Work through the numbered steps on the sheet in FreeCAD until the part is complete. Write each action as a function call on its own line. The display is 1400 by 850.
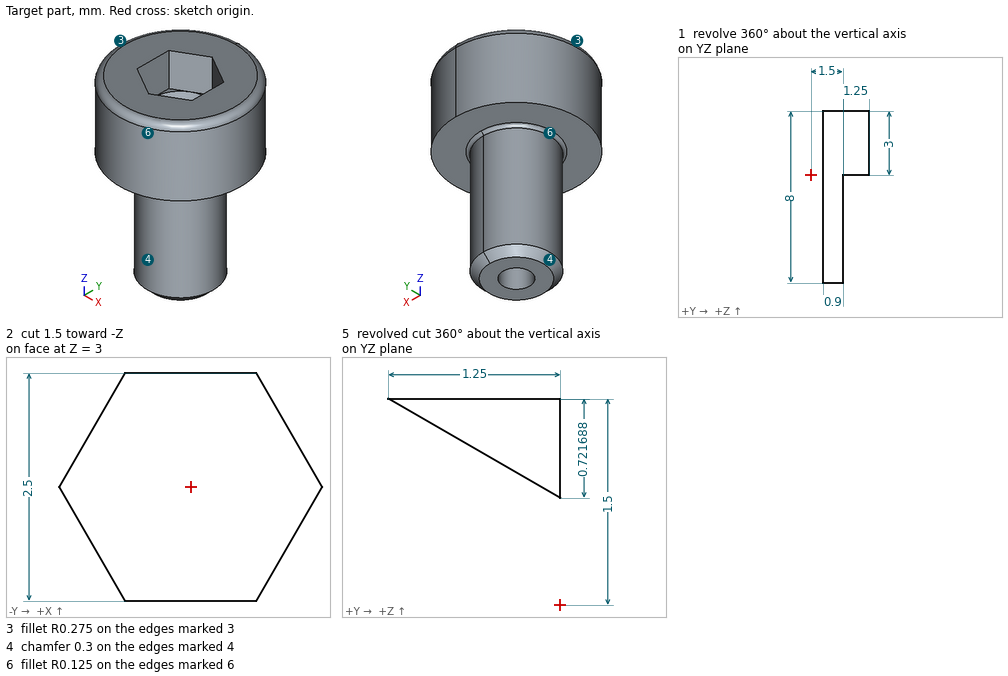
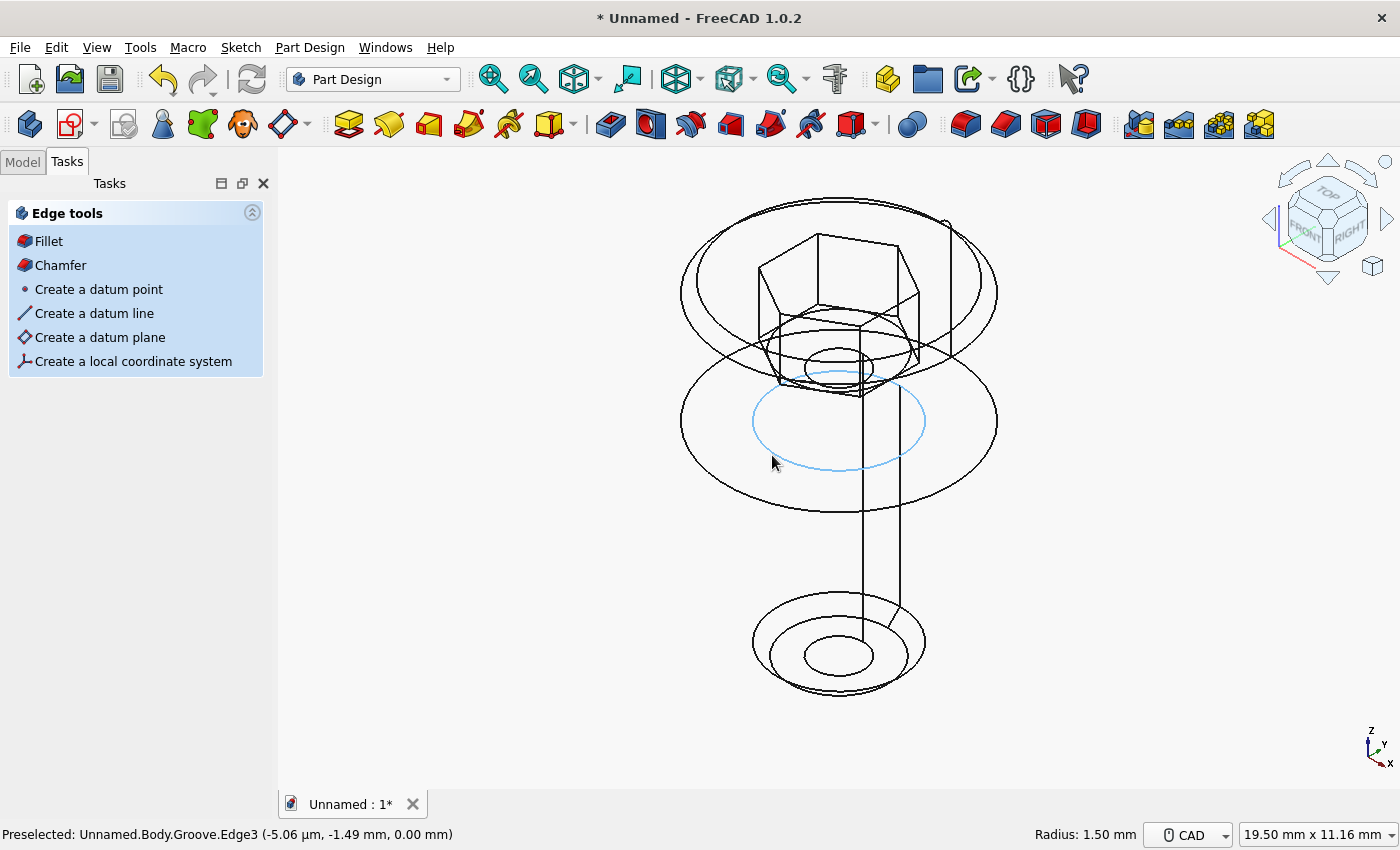
key(v)
key(1)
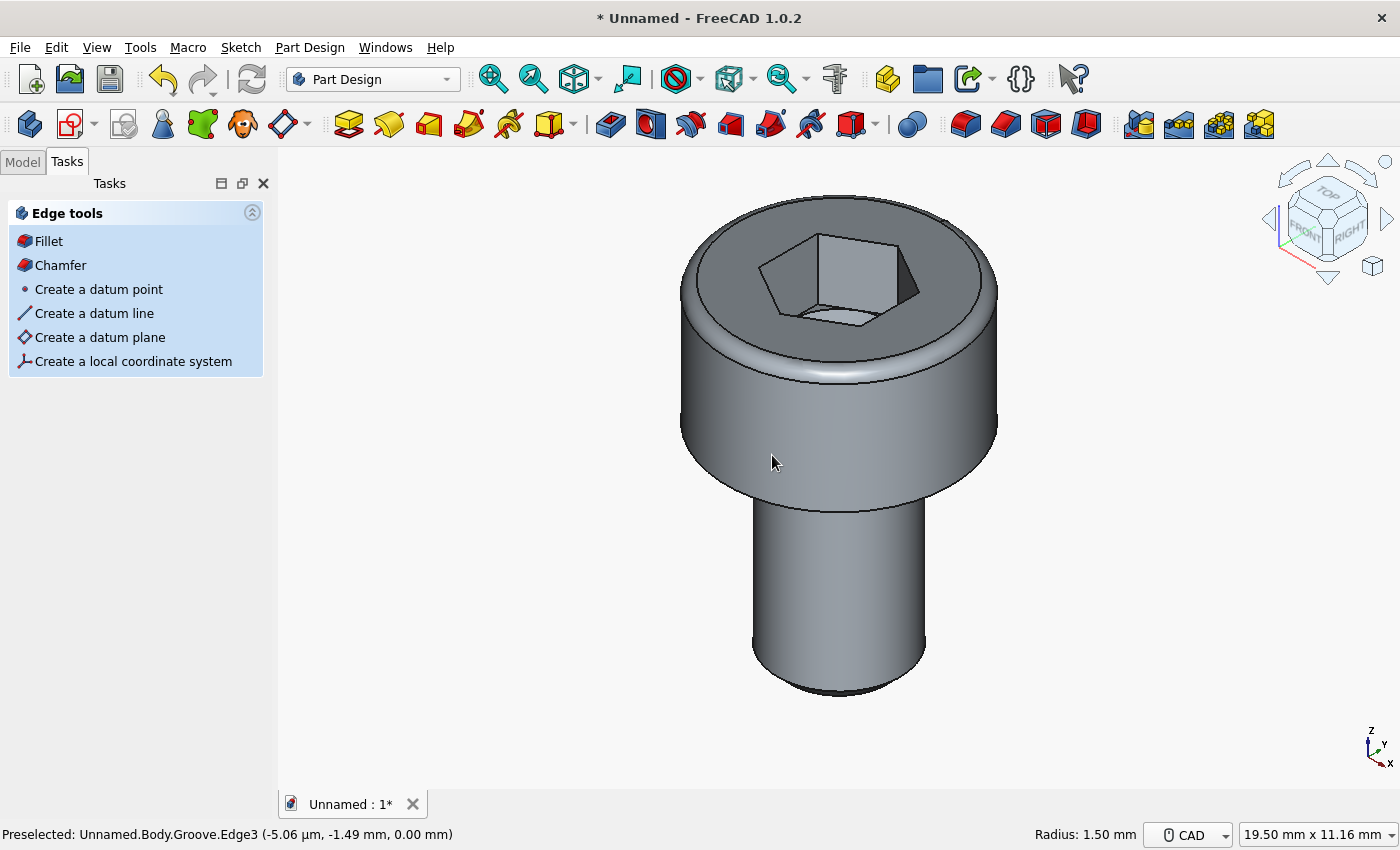
click(966, 124)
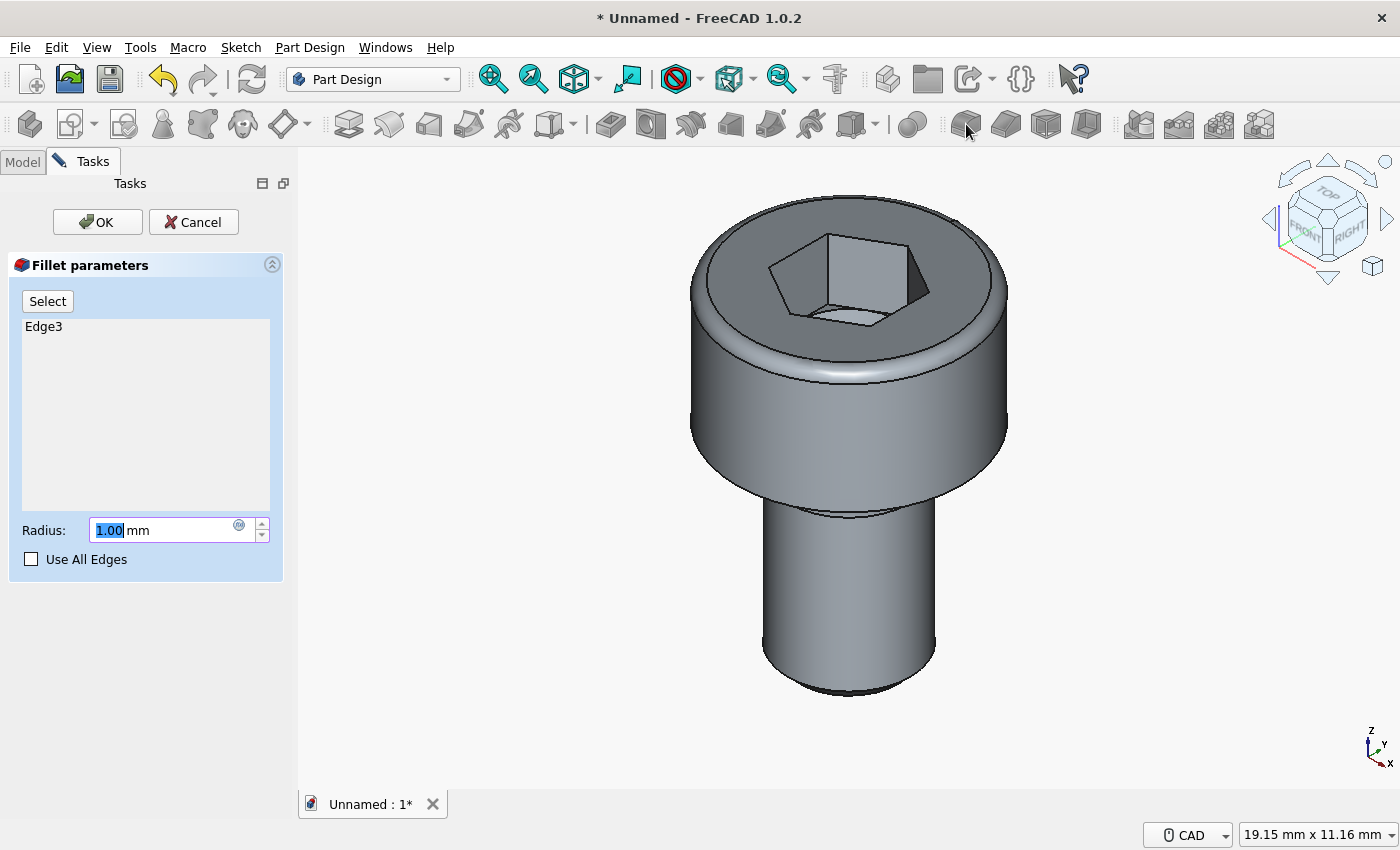
text(0.125)
key(Tab)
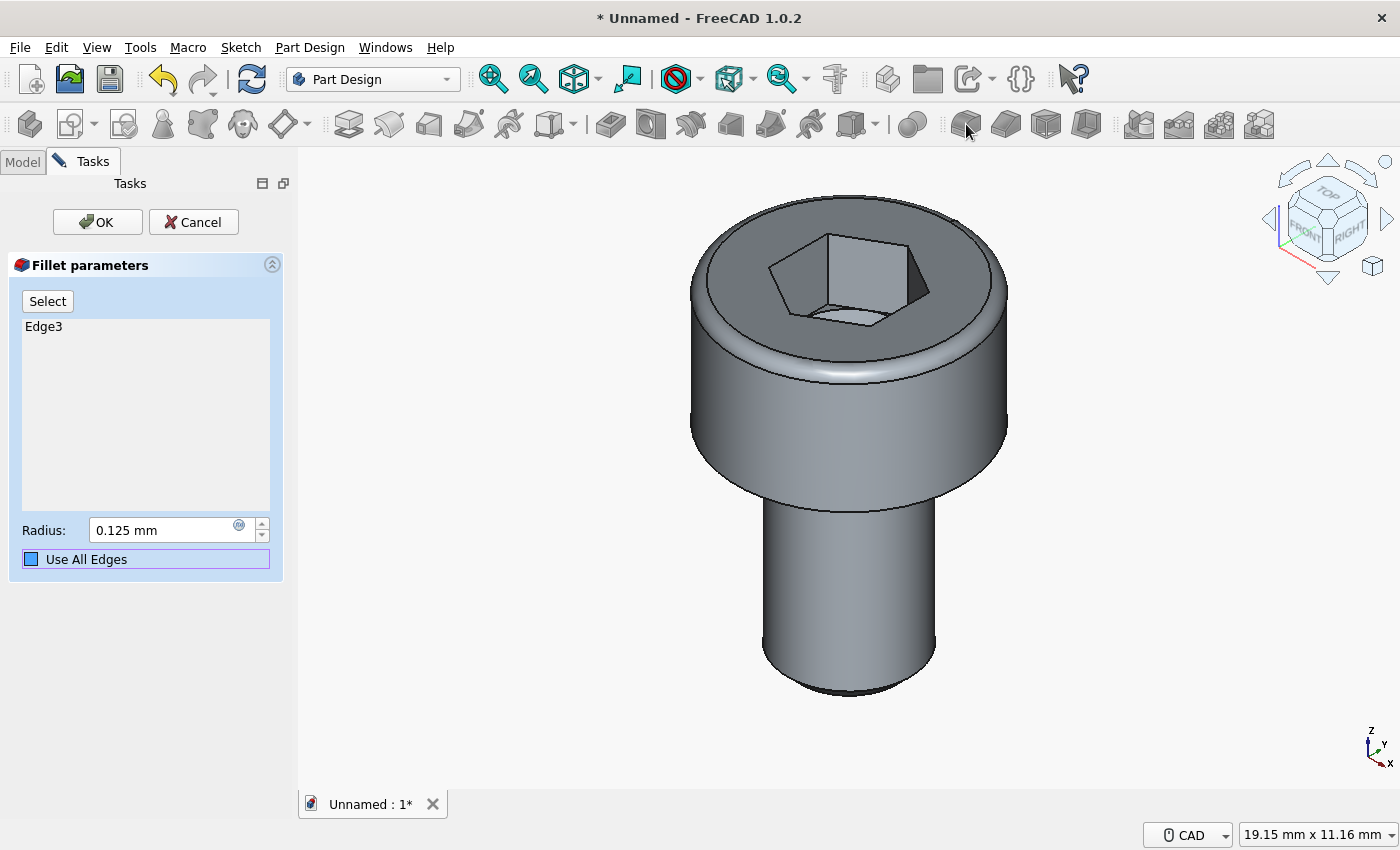
click(98, 222)